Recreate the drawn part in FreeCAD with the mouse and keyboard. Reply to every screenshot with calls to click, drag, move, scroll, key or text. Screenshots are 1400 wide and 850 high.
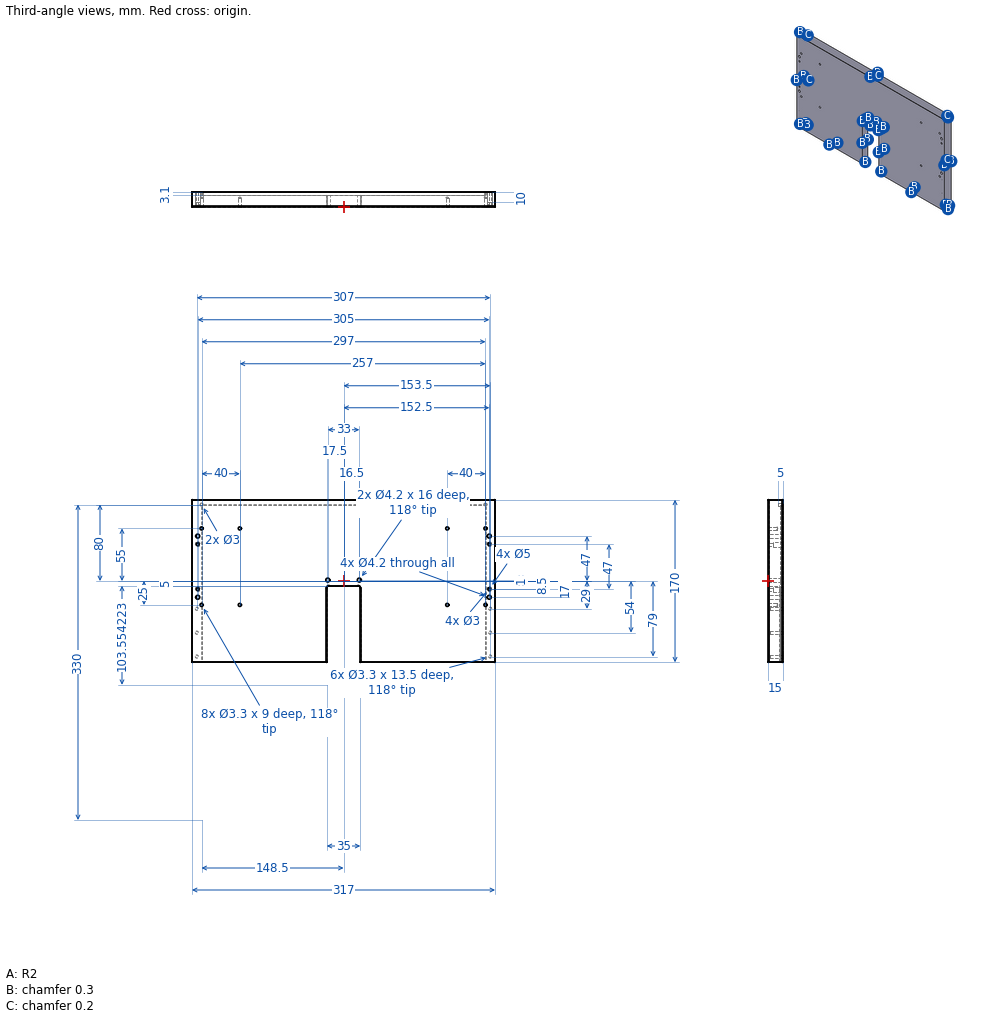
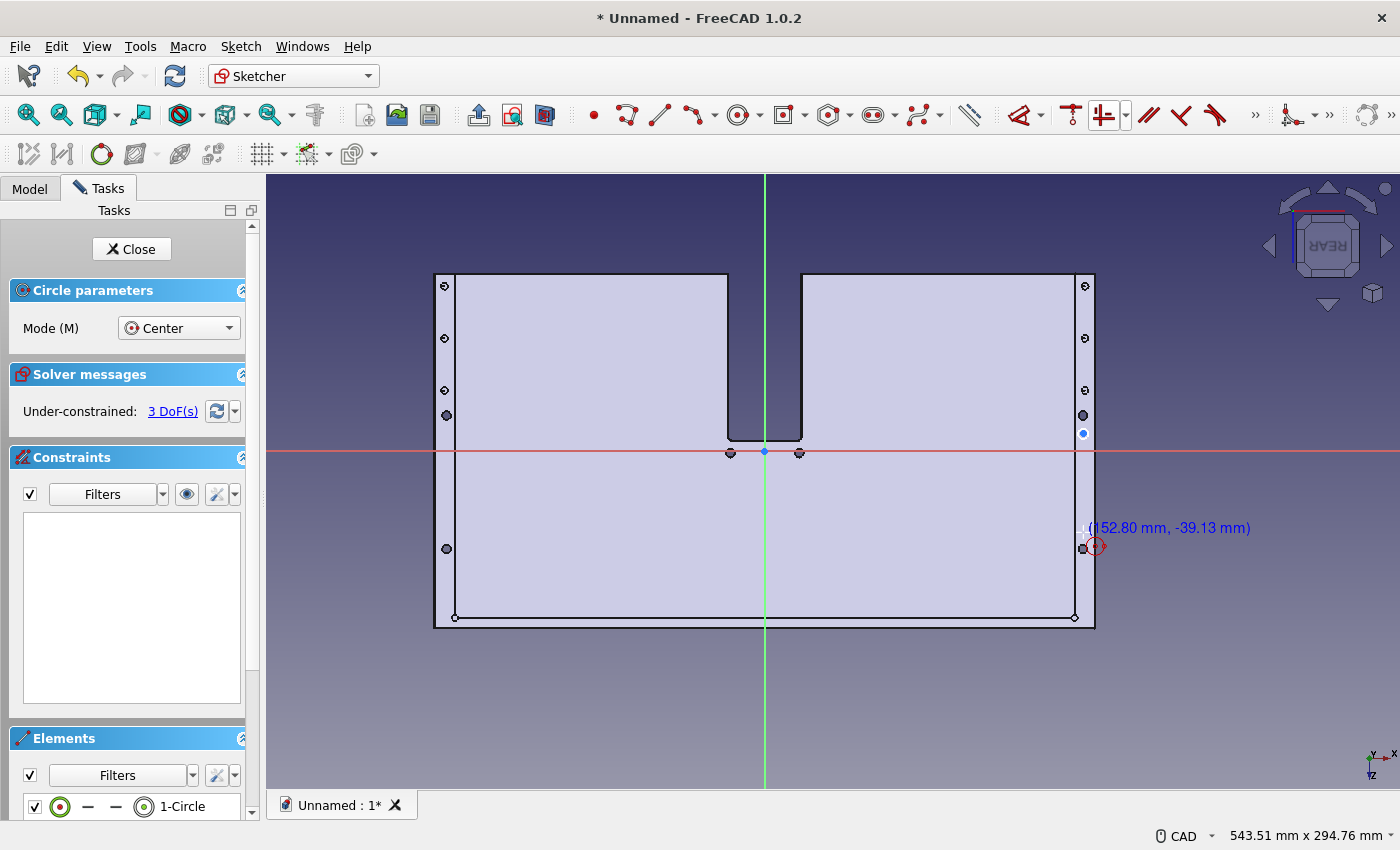
click(1083, 531)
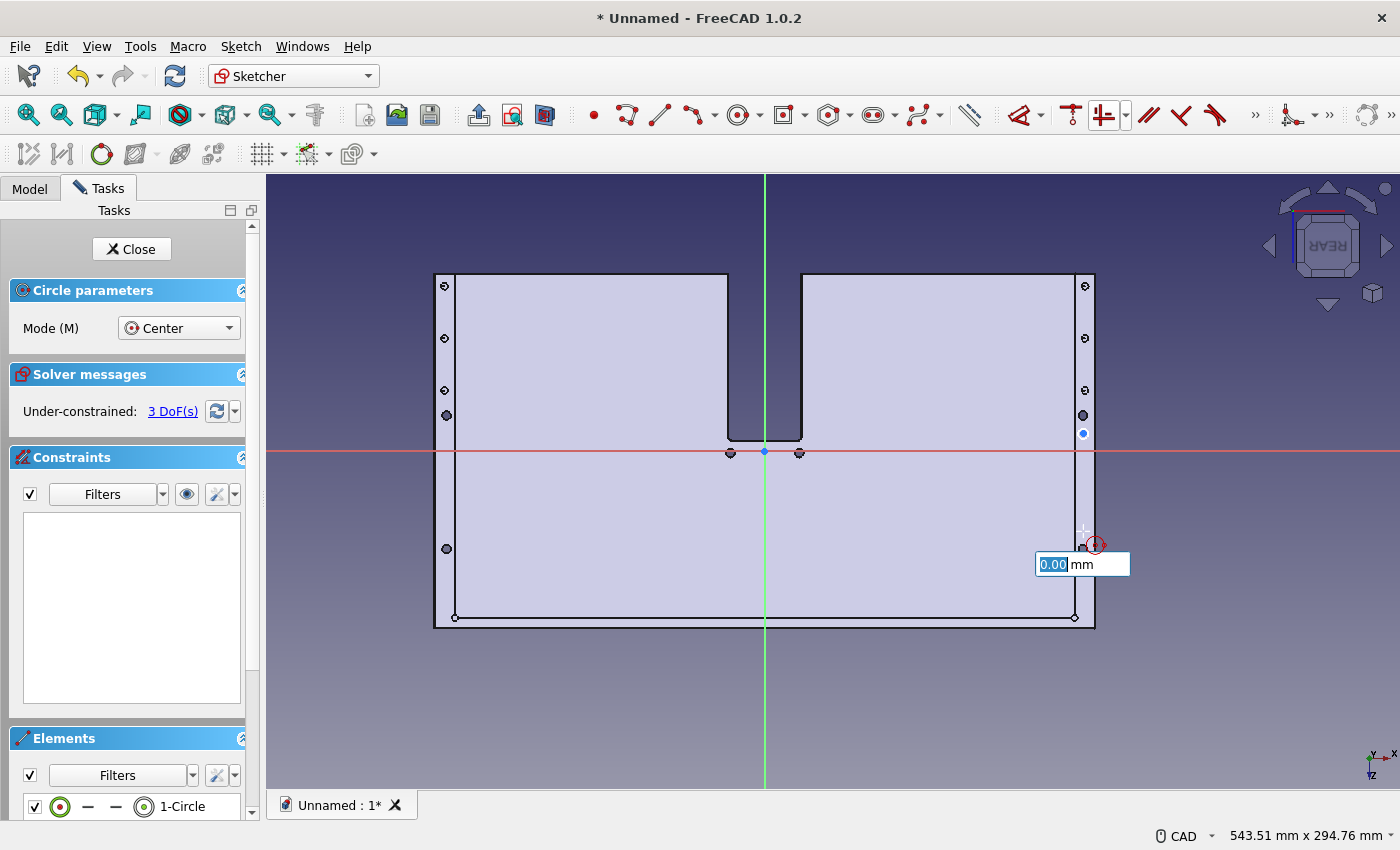
scroll(1087, 528, up, 6)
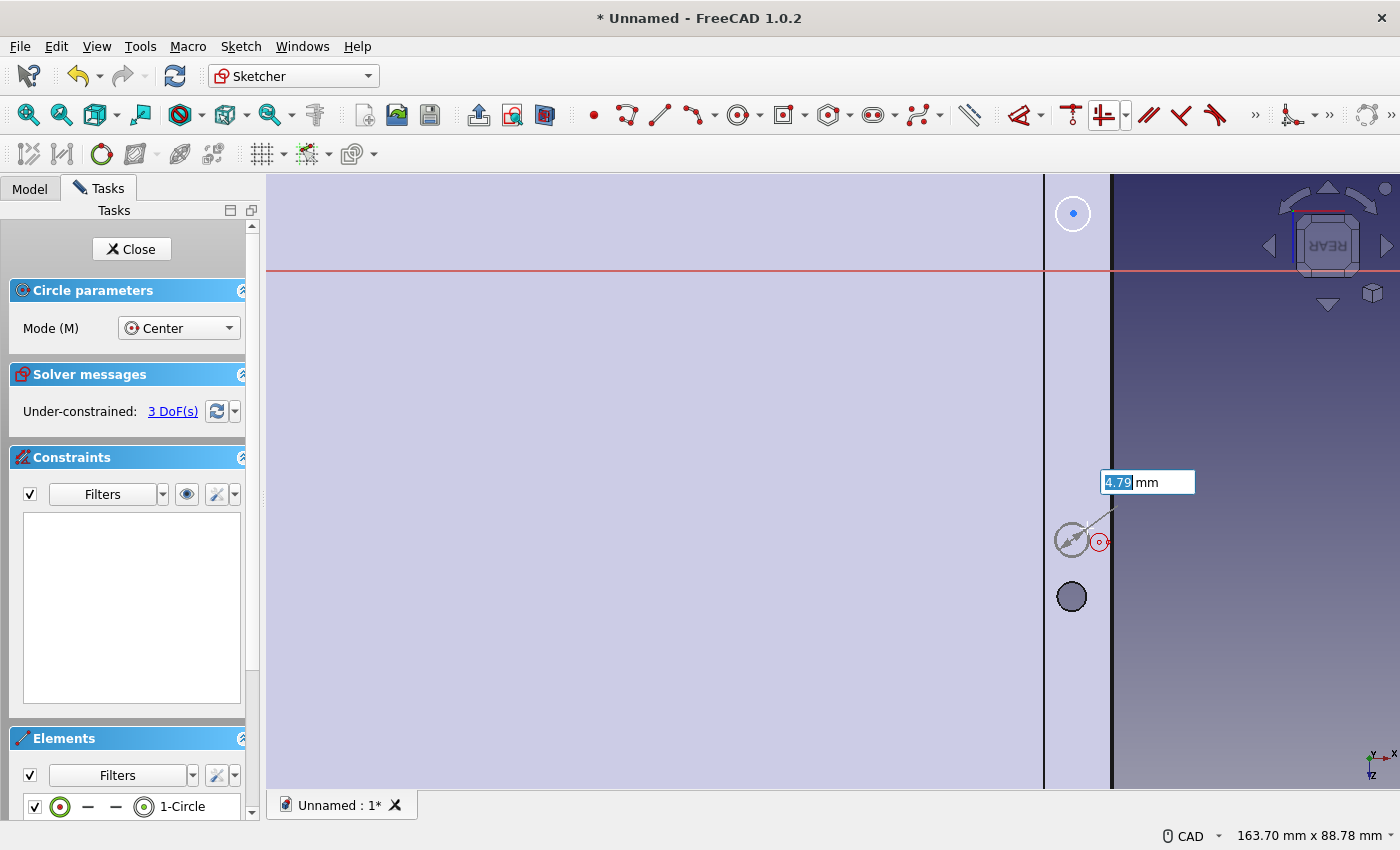
click(1084, 526)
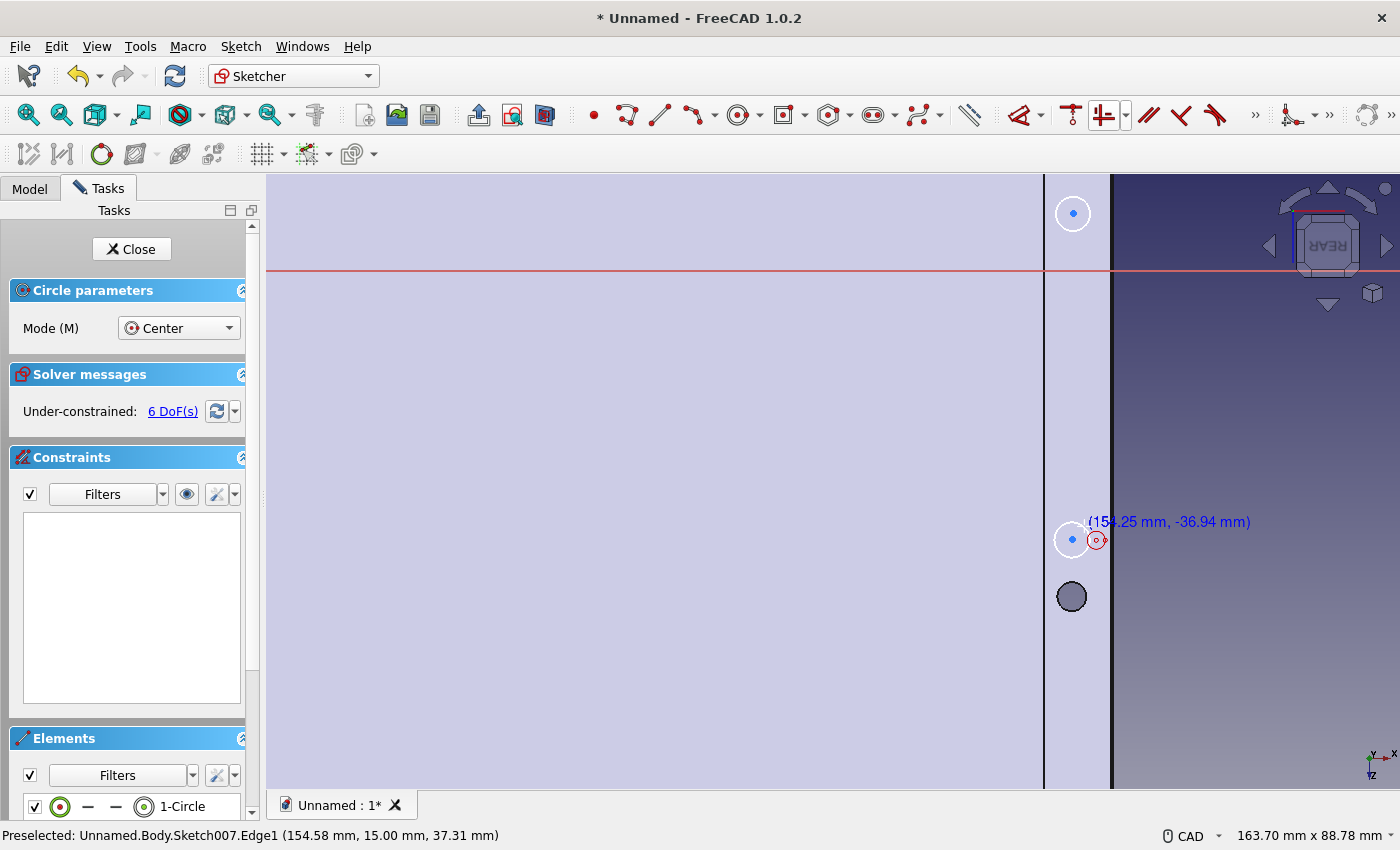
scroll(1087, 527, down, 6)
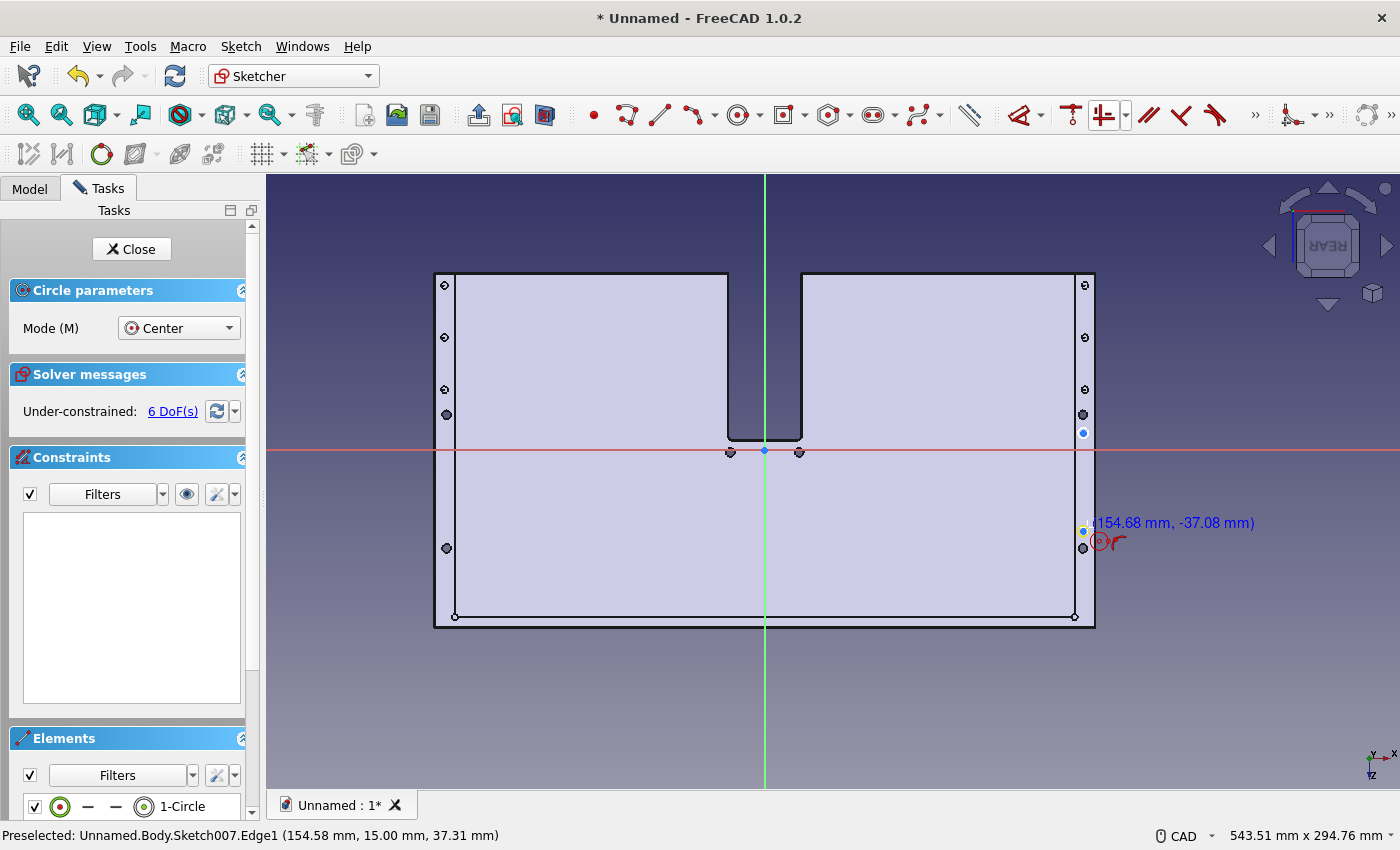
scroll(447, 433, up, 8)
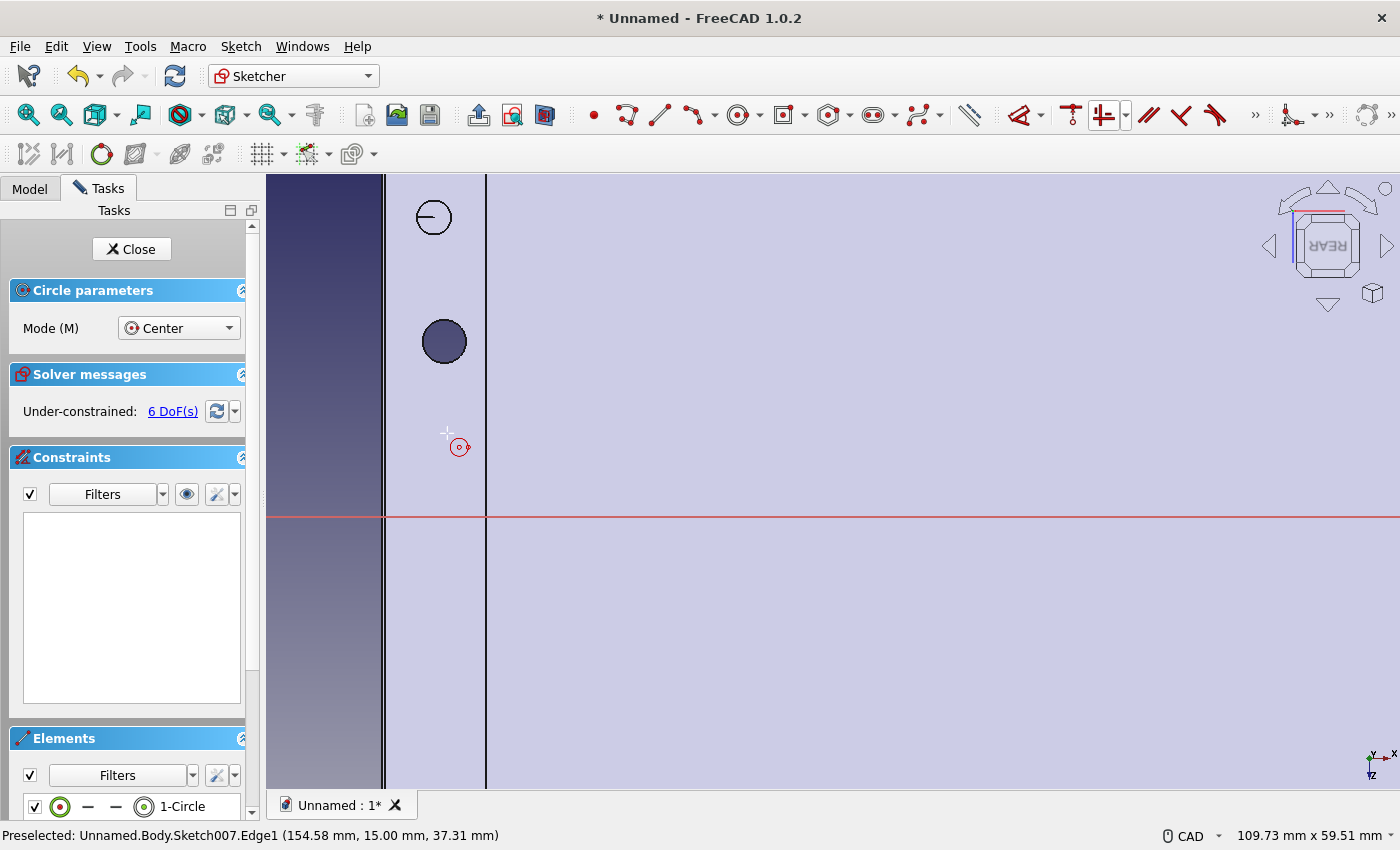
scroll(447, 433, down, 8)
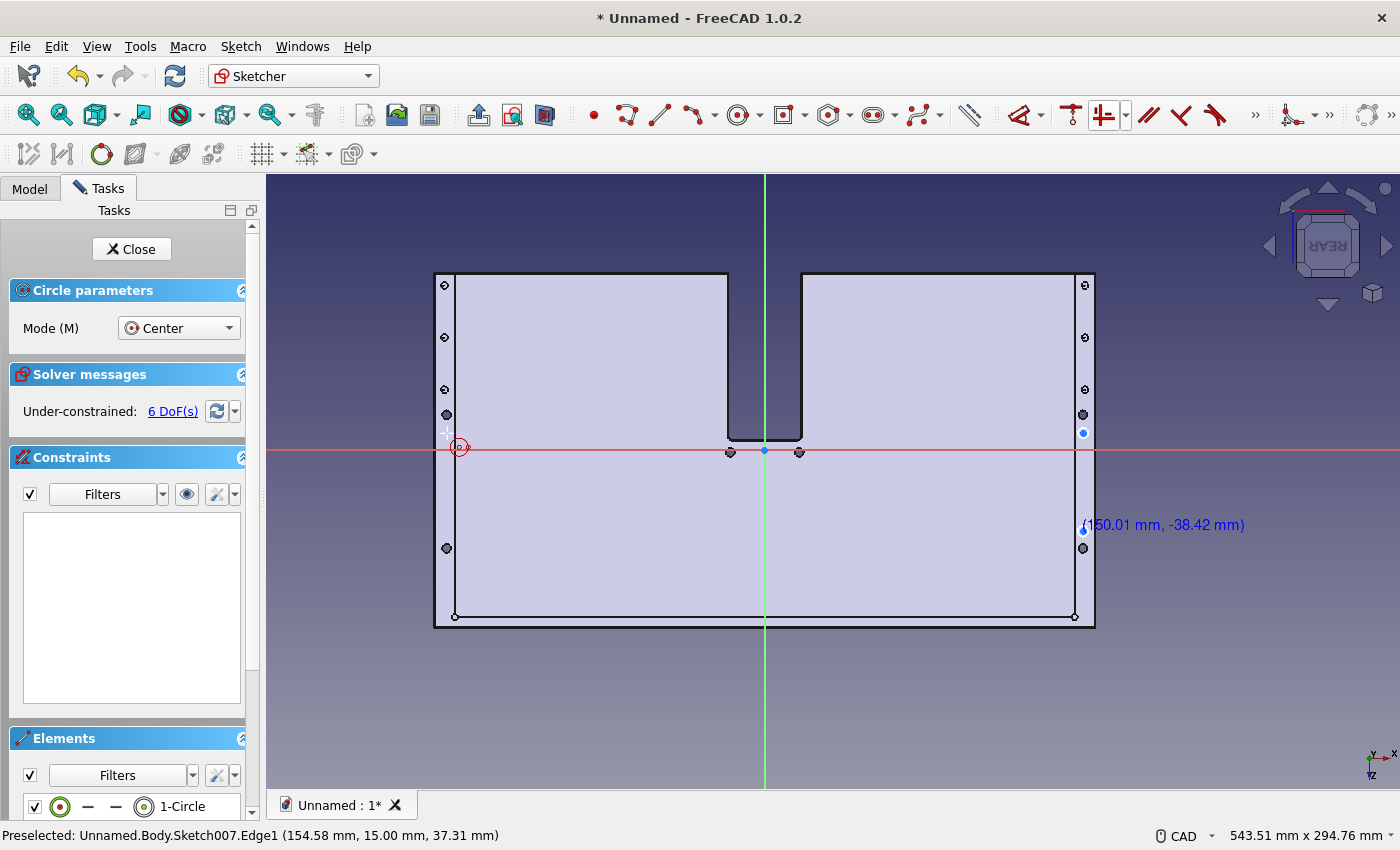
click(447, 433)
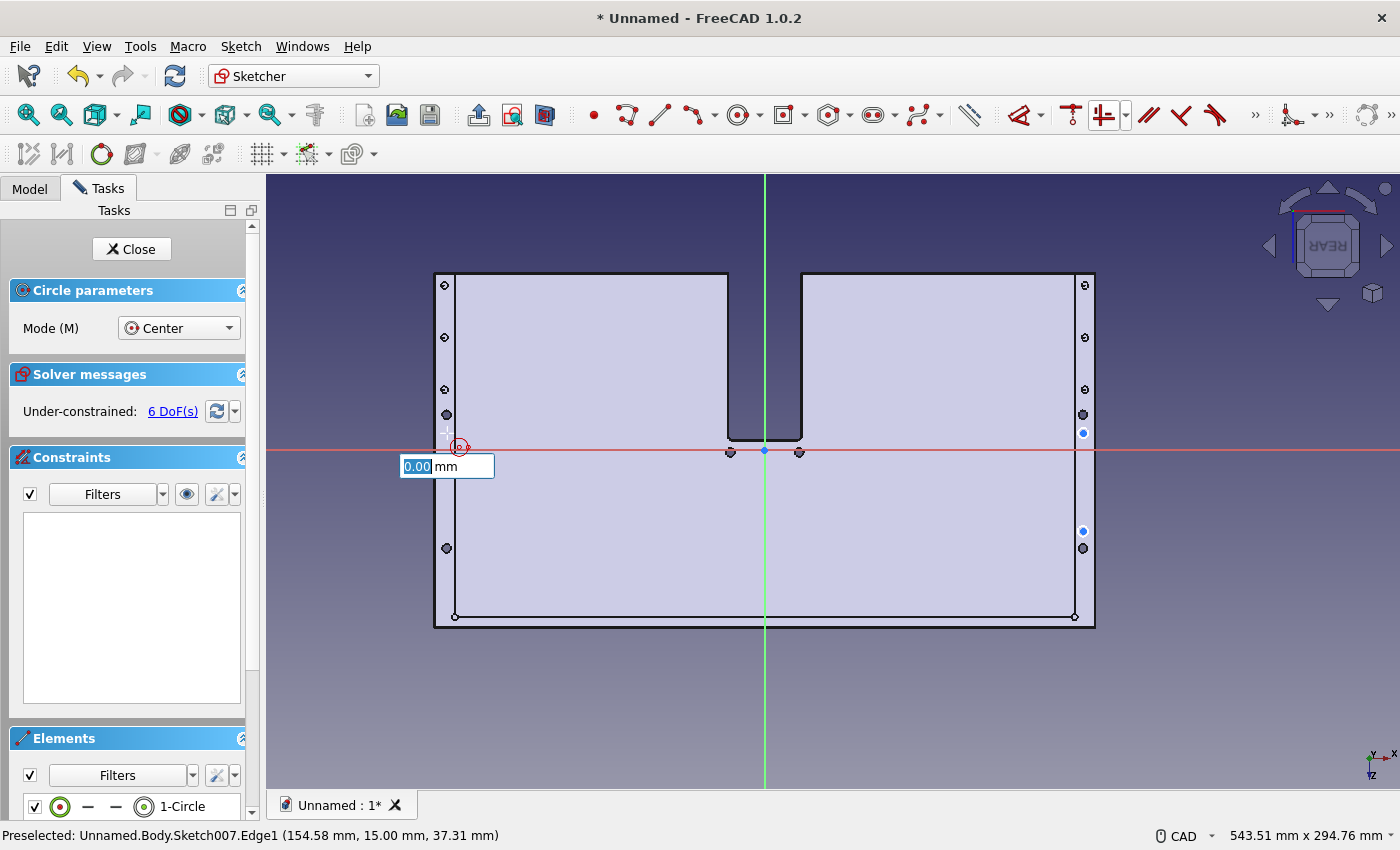
scroll(450, 429, up, 6)